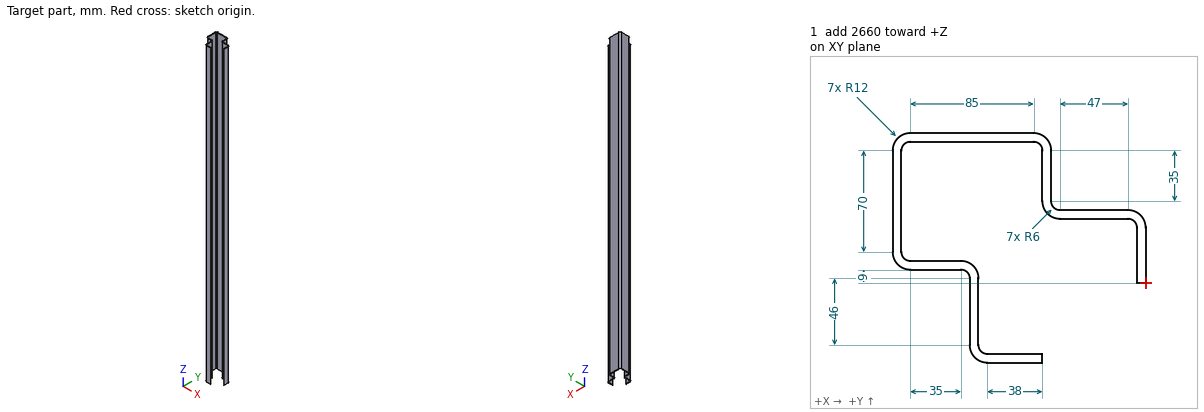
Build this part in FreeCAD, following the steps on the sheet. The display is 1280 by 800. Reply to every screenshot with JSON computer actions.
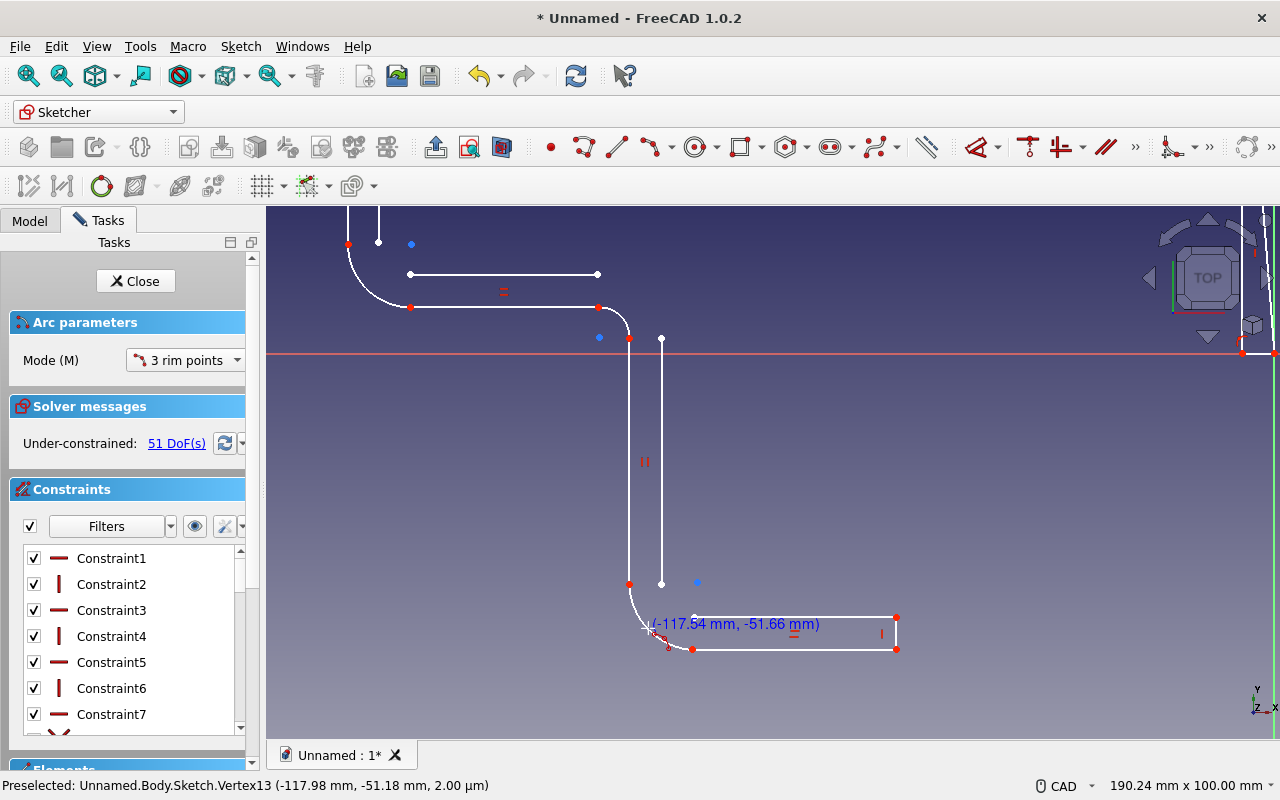
{"action": "left_click", "coordinate": [694, 617]}
{"action": "left_click", "coordinate": [662, 584]}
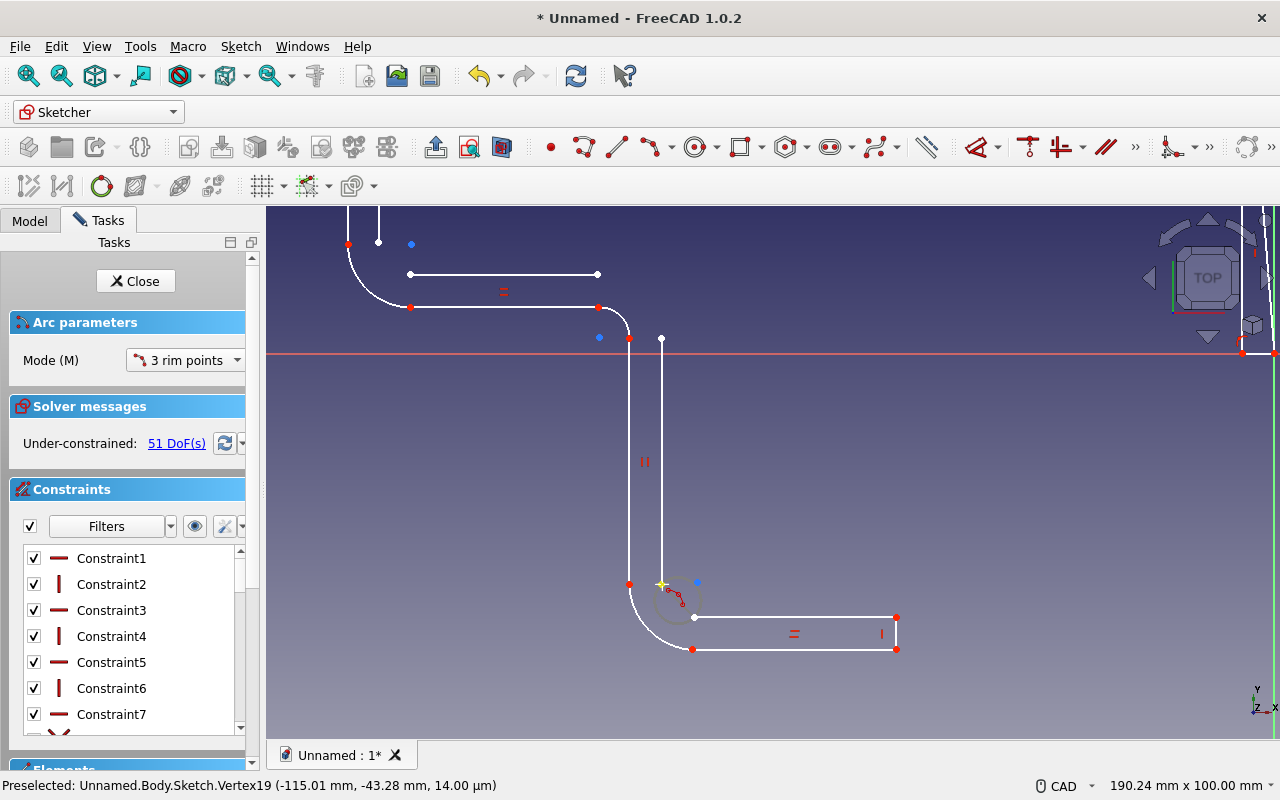
{"action": "scroll", "coordinate": [671, 605], "scroll_direction": "up", "scroll_amount": 3}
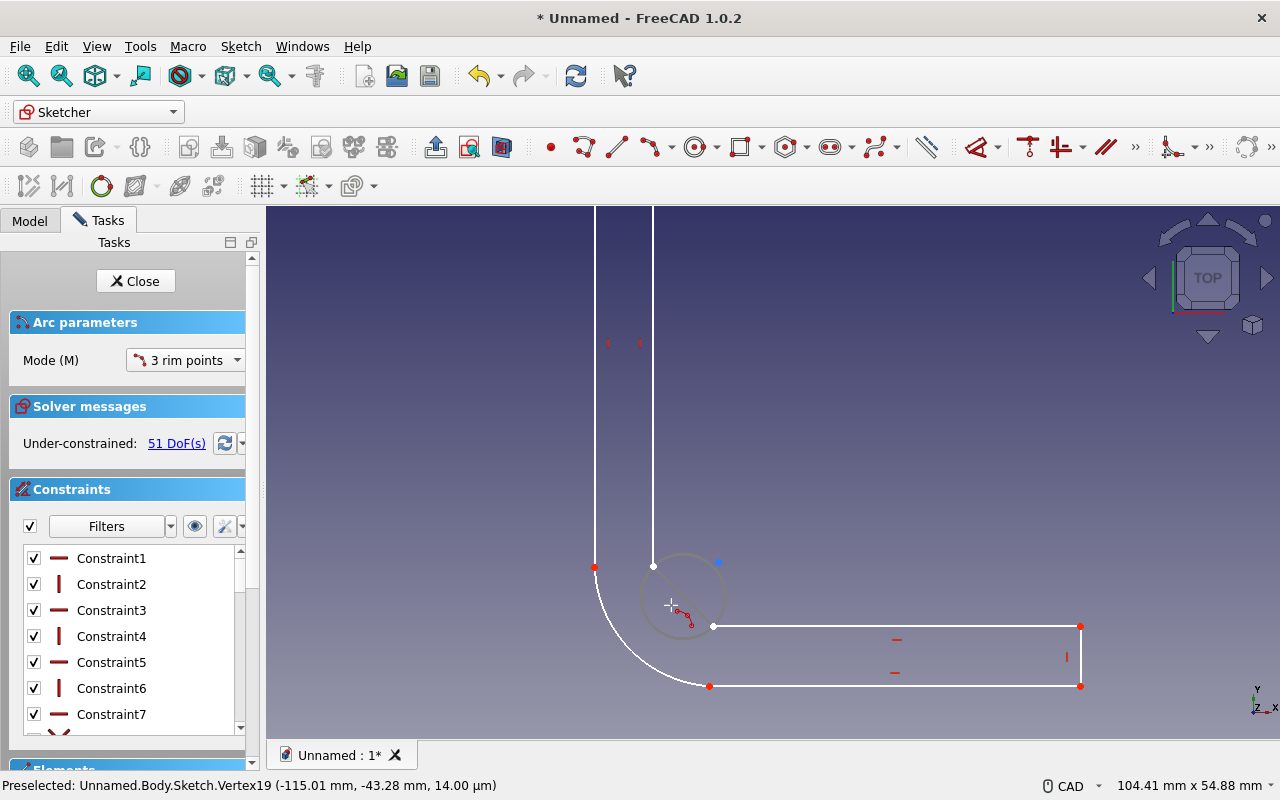
{"action": "left_click", "coordinate": [671, 605]}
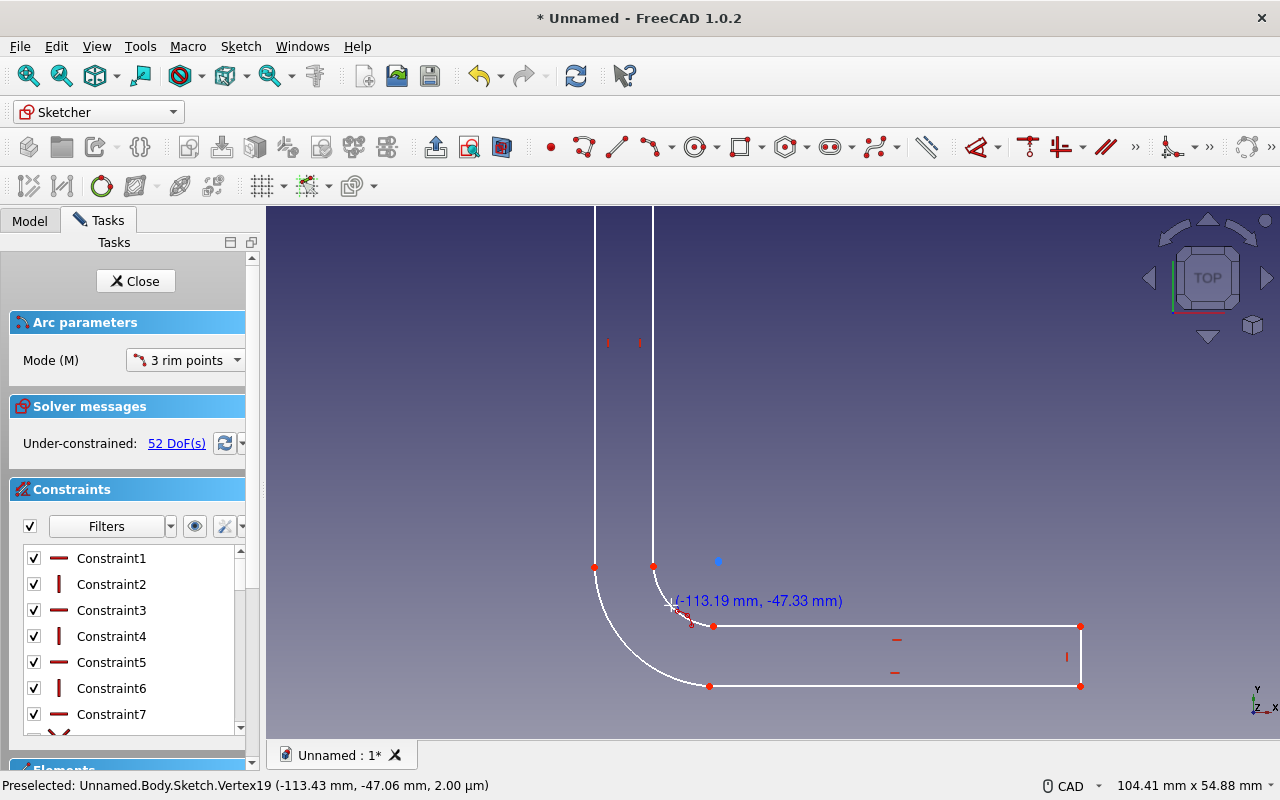
{"action": "scroll", "coordinate": [649, 614], "scroll_direction": "down", "scroll_amount": 8}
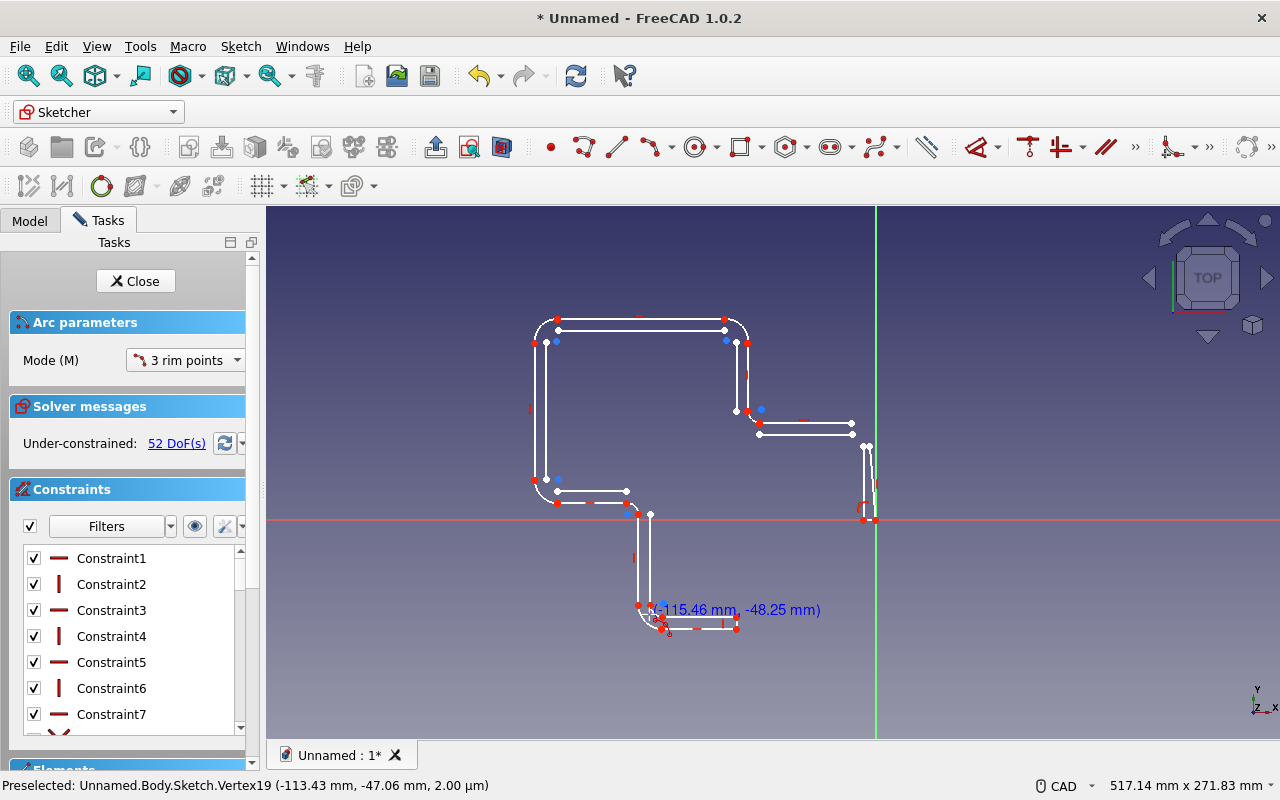
{"action": "scroll", "coordinate": [650, 514], "scroll_direction": "up", "scroll_amount": 5}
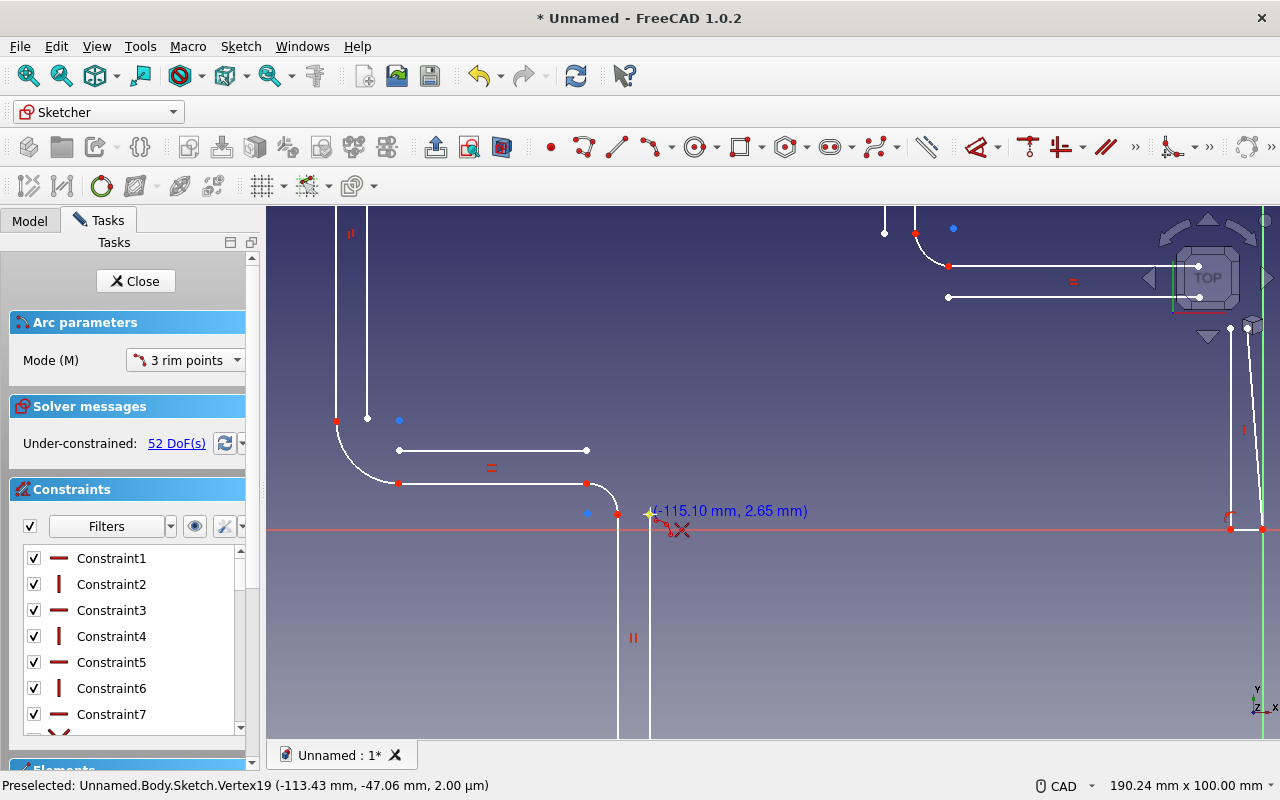
{"action": "left_click", "coordinate": [650, 515]}
{"action": "left_click", "coordinate": [586, 451]}
{"action": "left_click", "coordinate": [631, 469]}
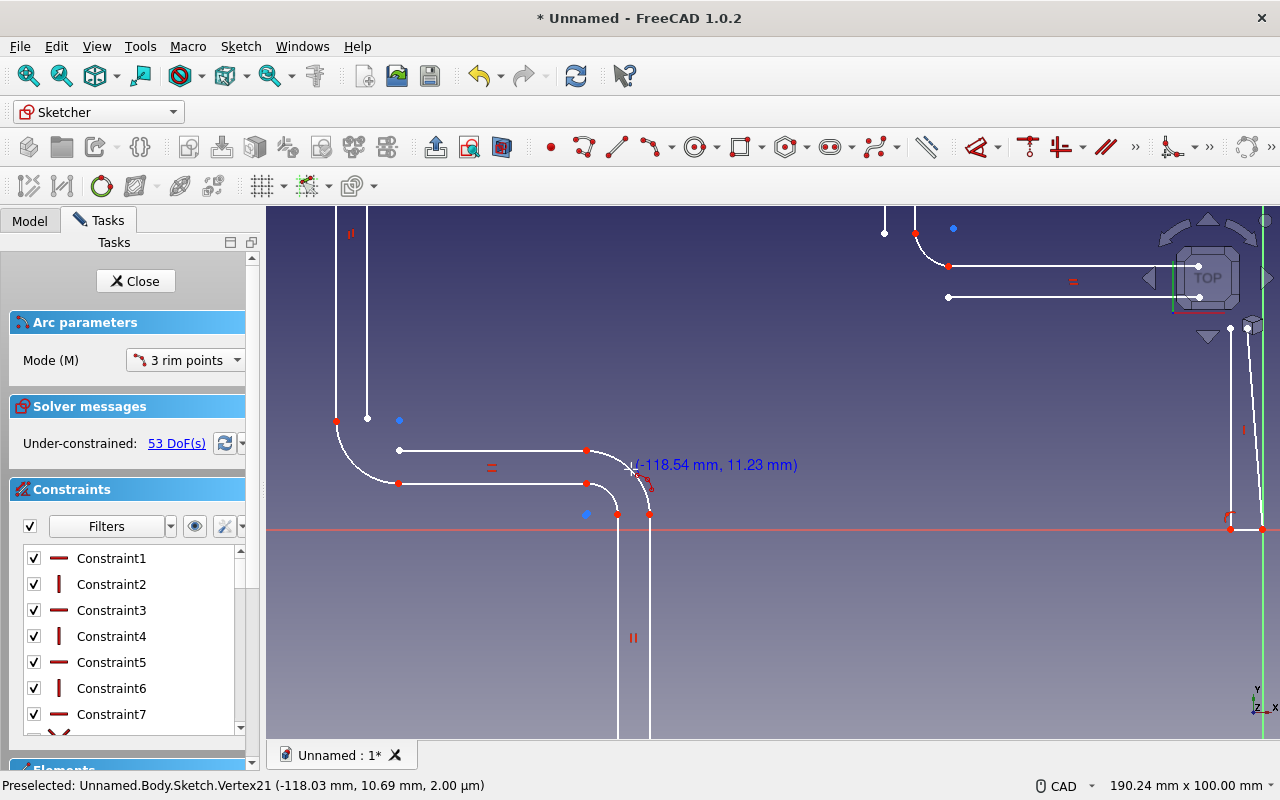
{"action": "left_click", "coordinate": [399, 451]}
{"action": "left_click", "coordinate": [367, 419]}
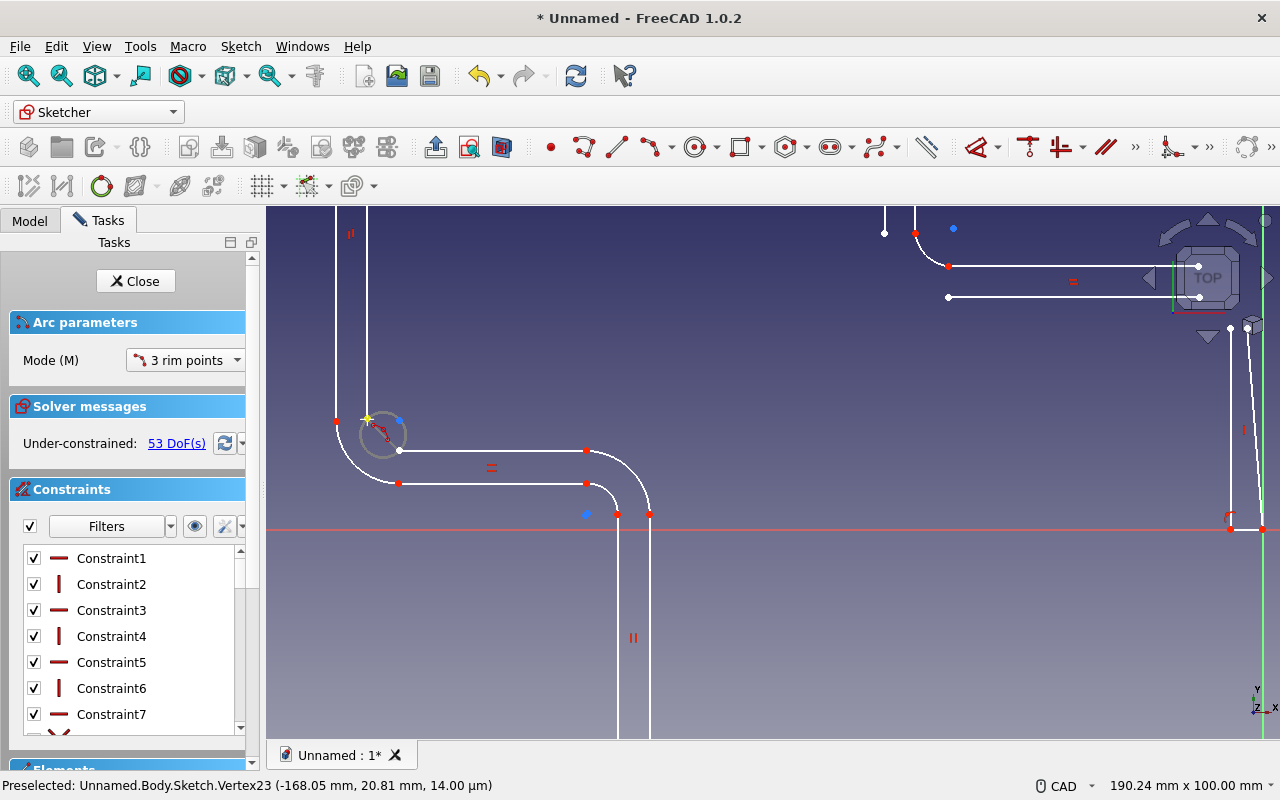
{"action": "scroll", "coordinate": [377, 441], "scroll_direction": "up", "scroll_amount": 3}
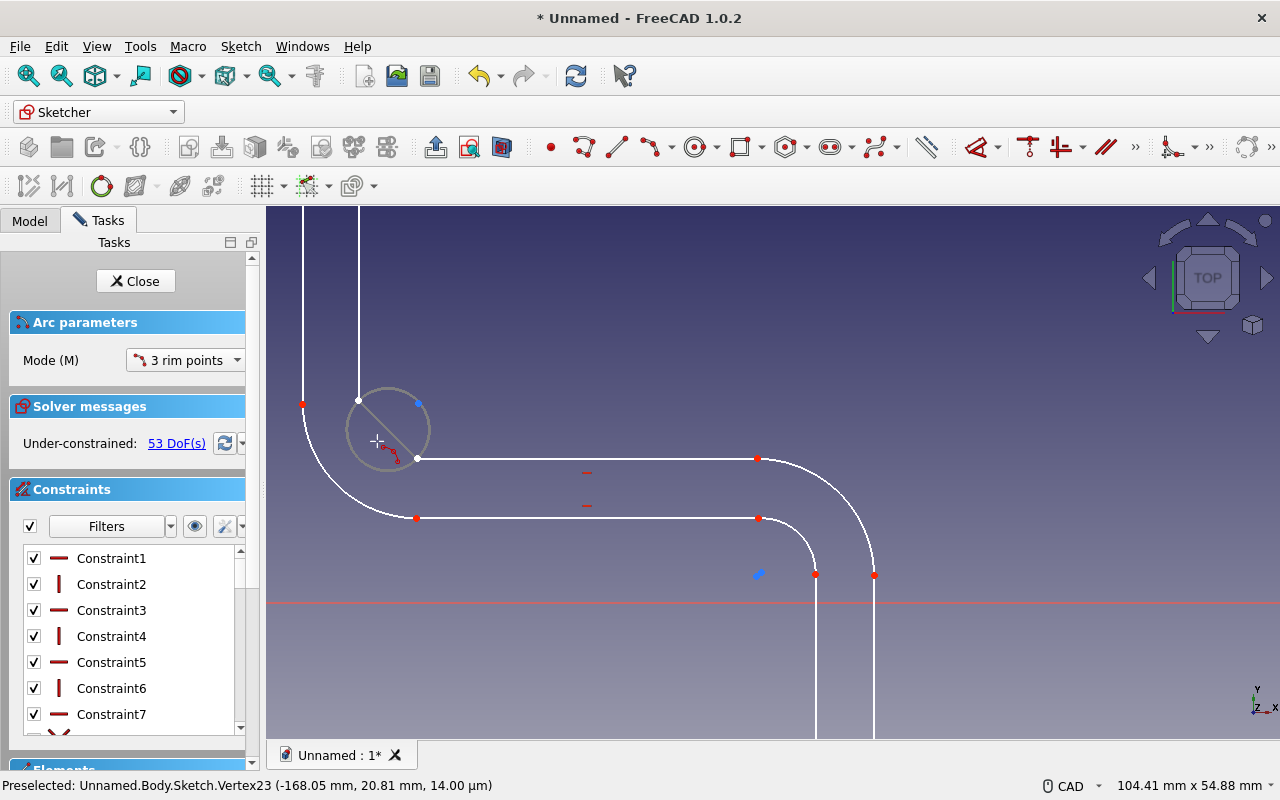
{"action": "left_click", "coordinate": [376, 440]}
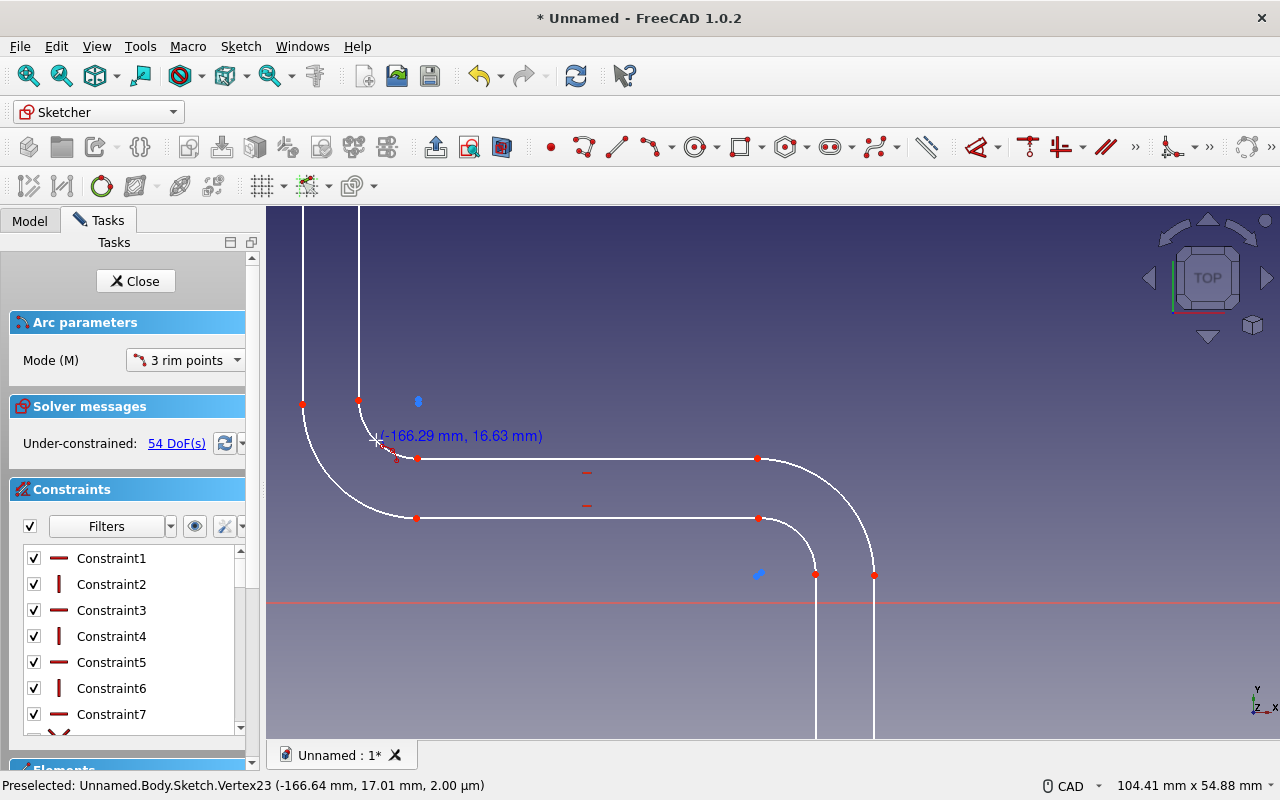
{"action": "scroll", "coordinate": [593, 499], "scroll_direction": "down", "scroll_amount": 8}